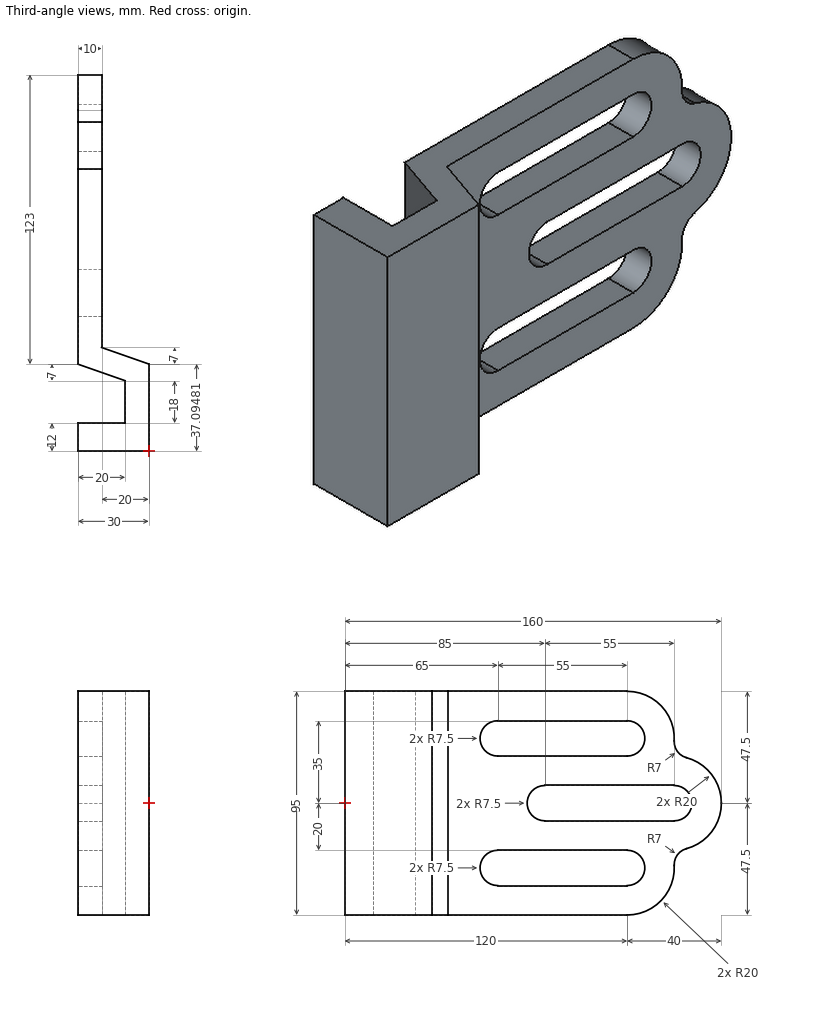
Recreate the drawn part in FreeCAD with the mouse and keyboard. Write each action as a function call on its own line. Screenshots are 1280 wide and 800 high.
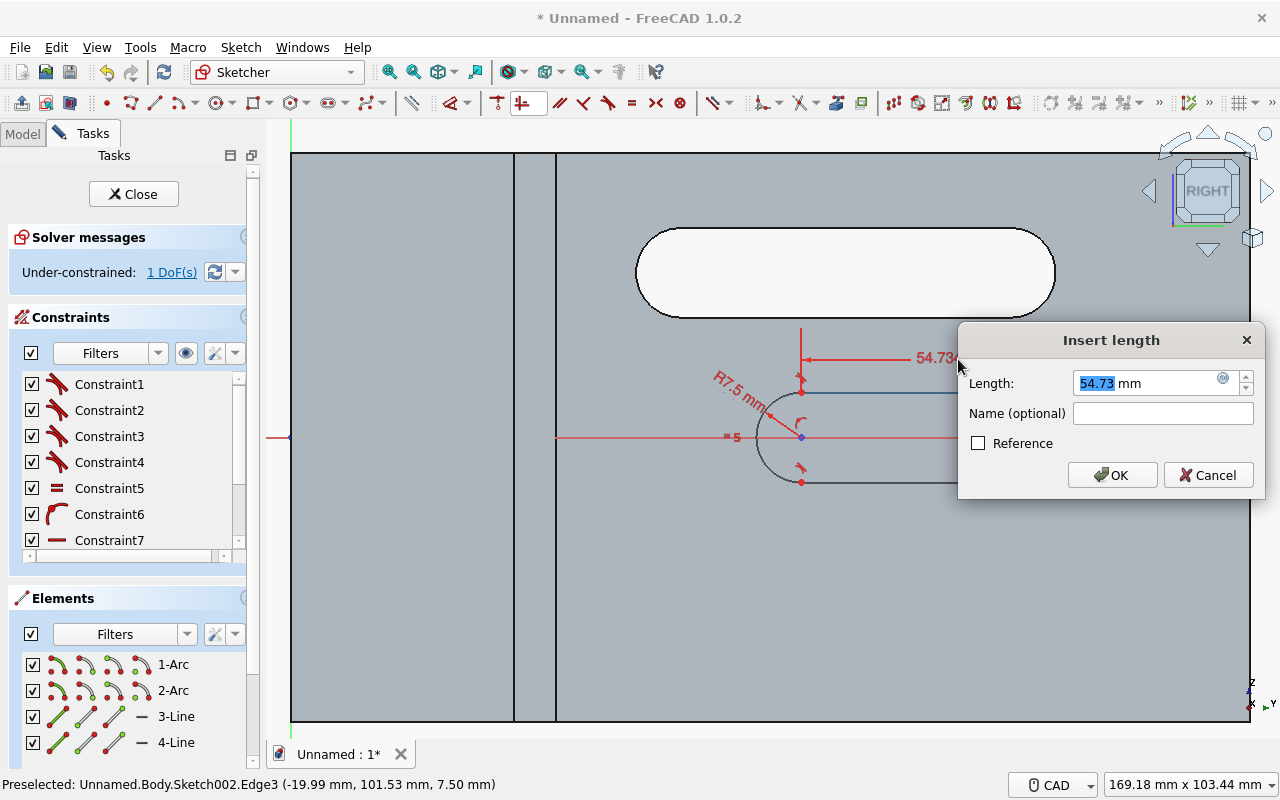
text(55)
key(Return)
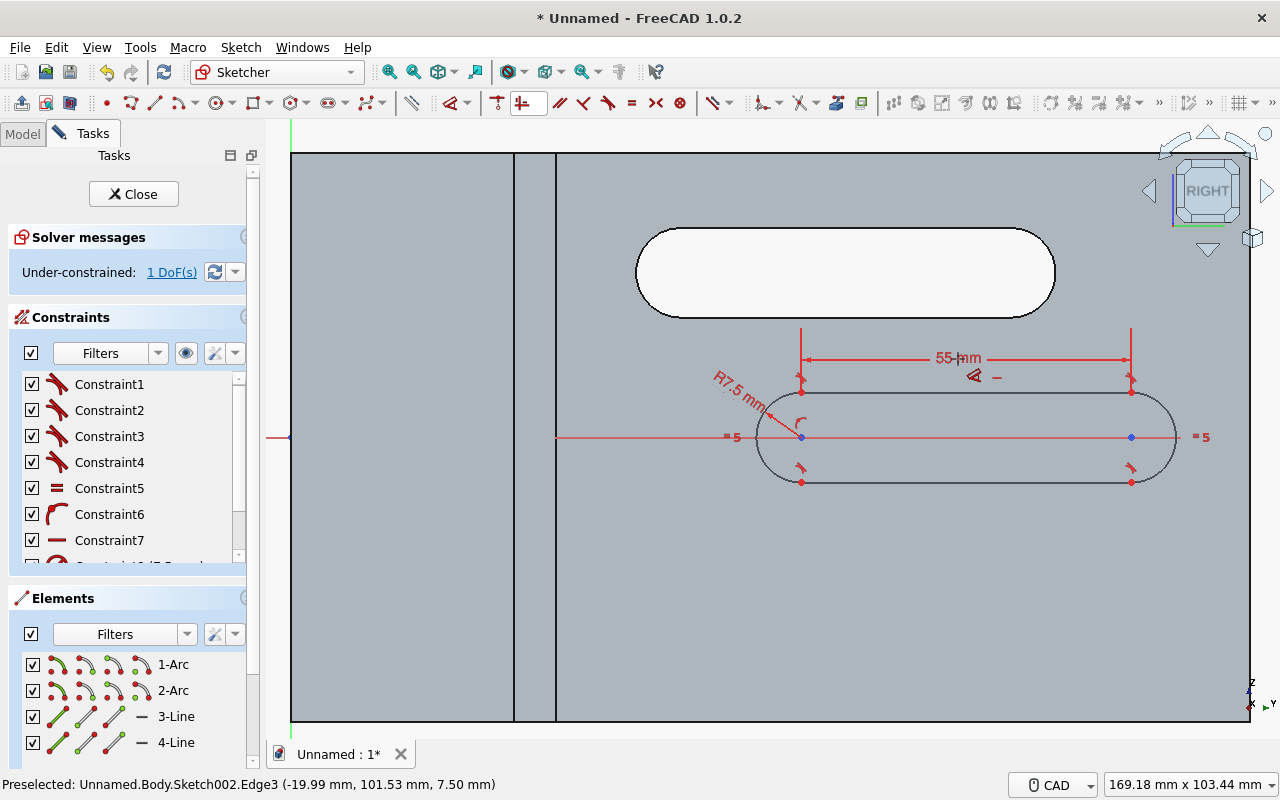
click(801, 393)
click(548, 359)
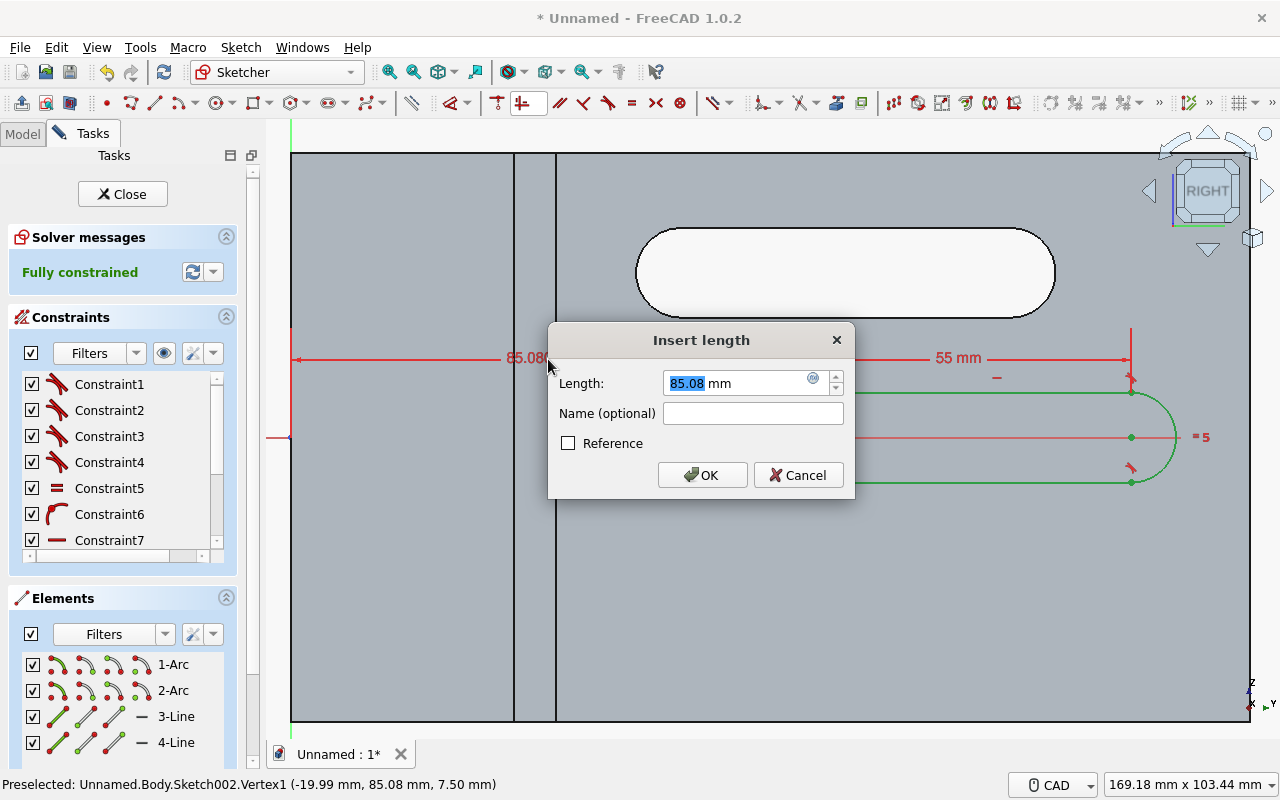
text(85)
key(Return)
key(Escape)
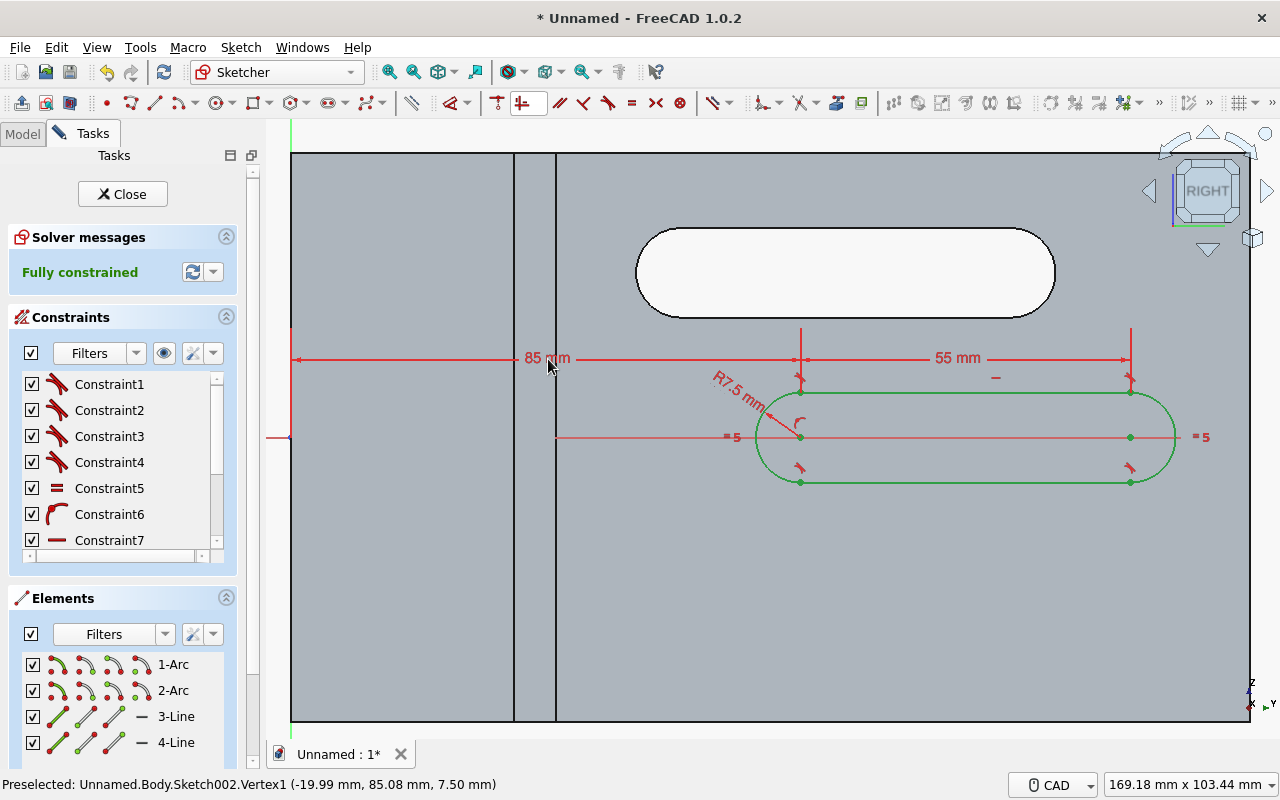
click(123, 194)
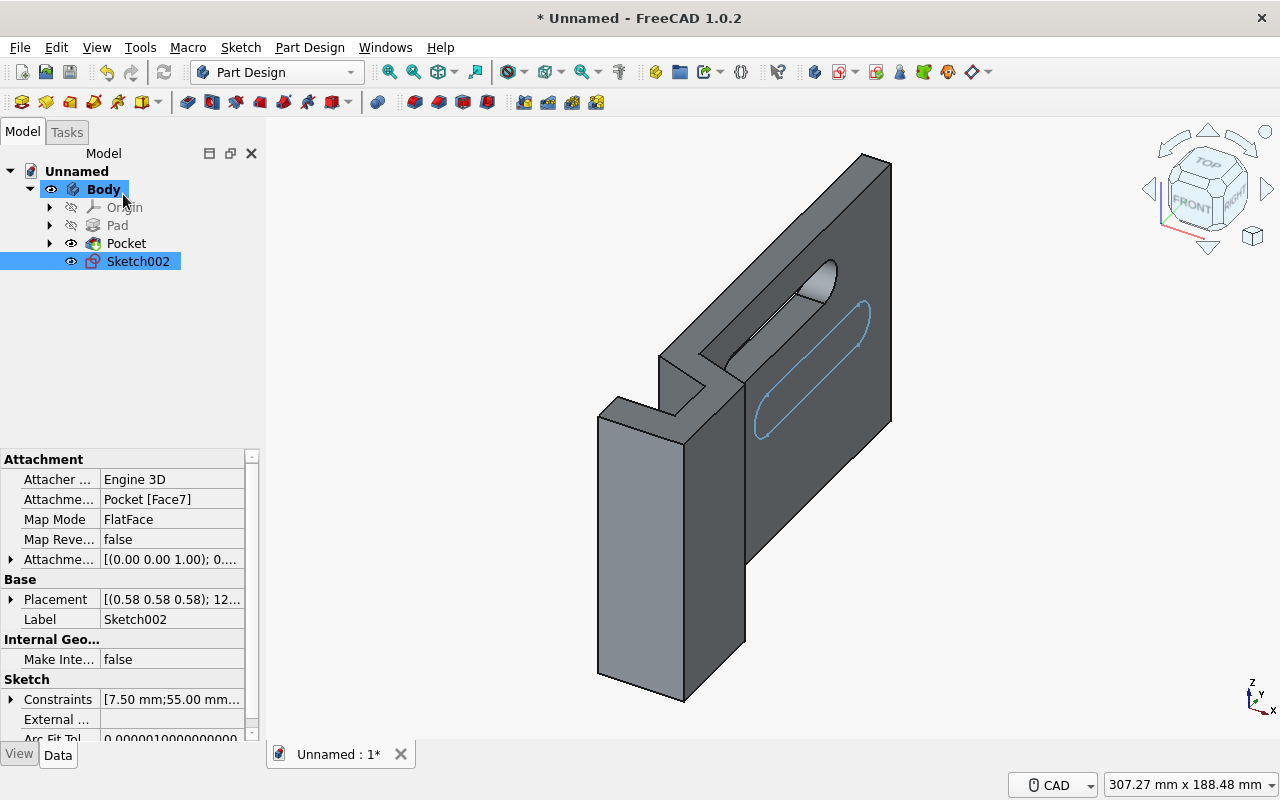
click(188, 102)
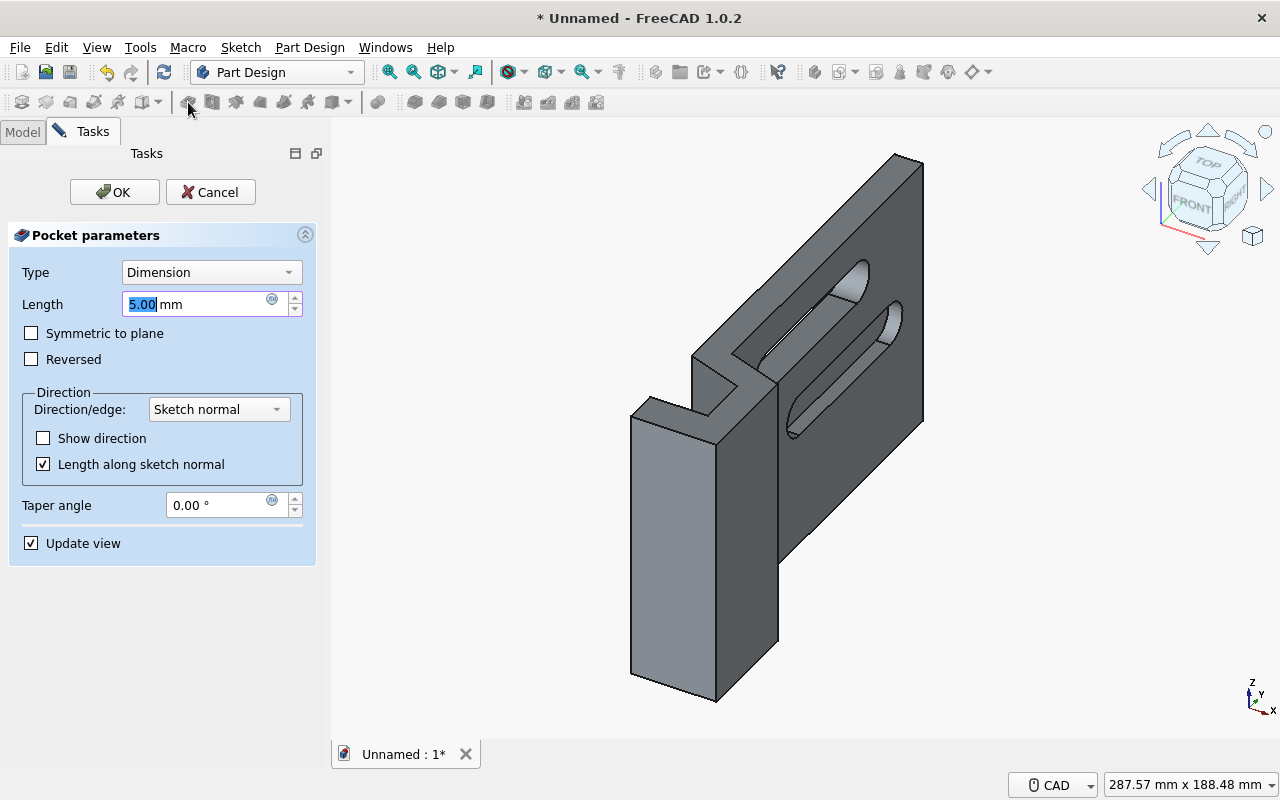
click(212, 272)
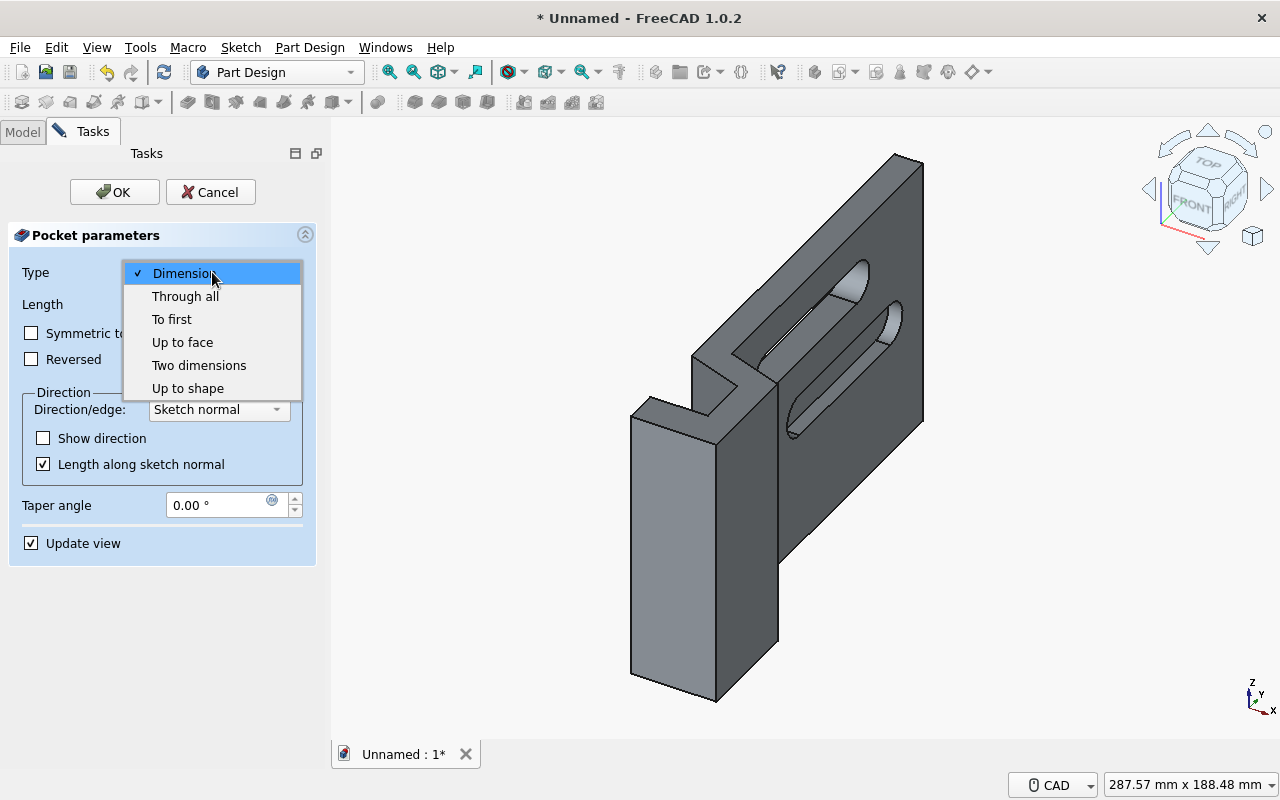
click(212, 320)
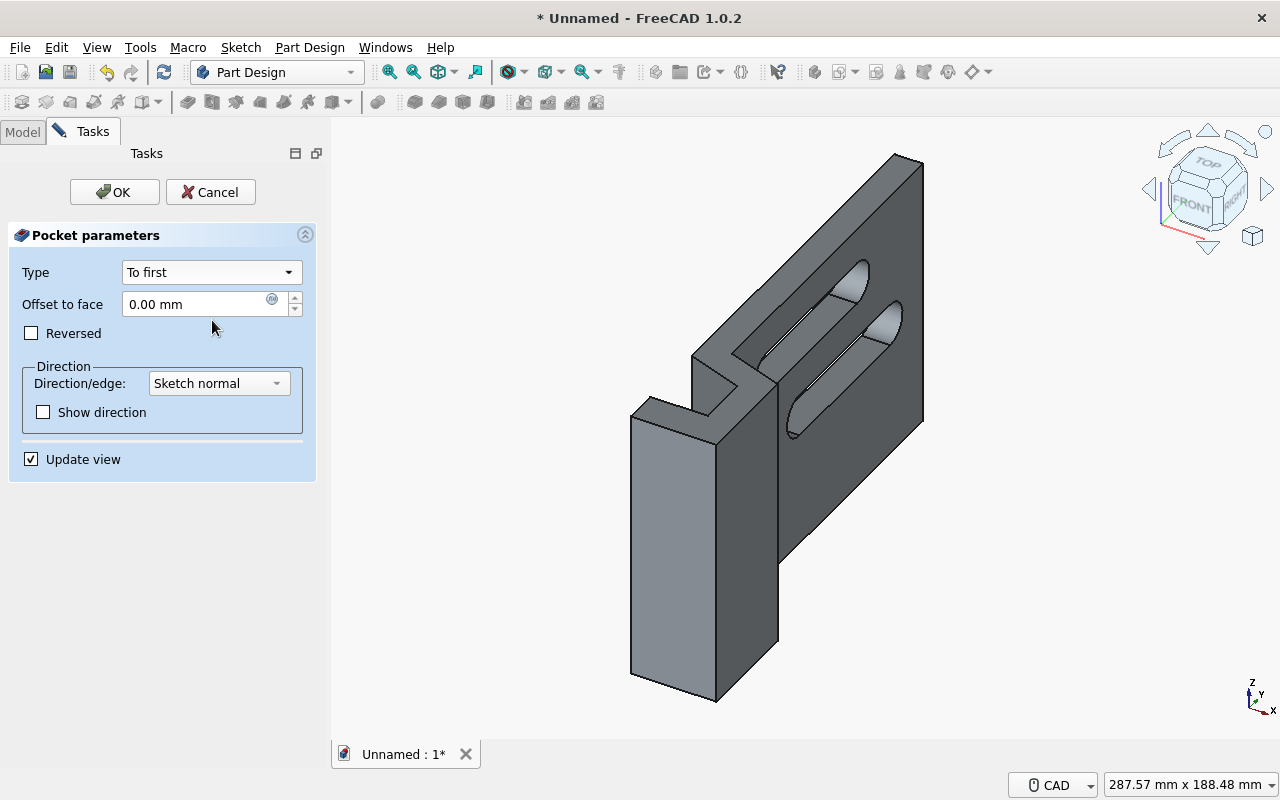
click(115, 192)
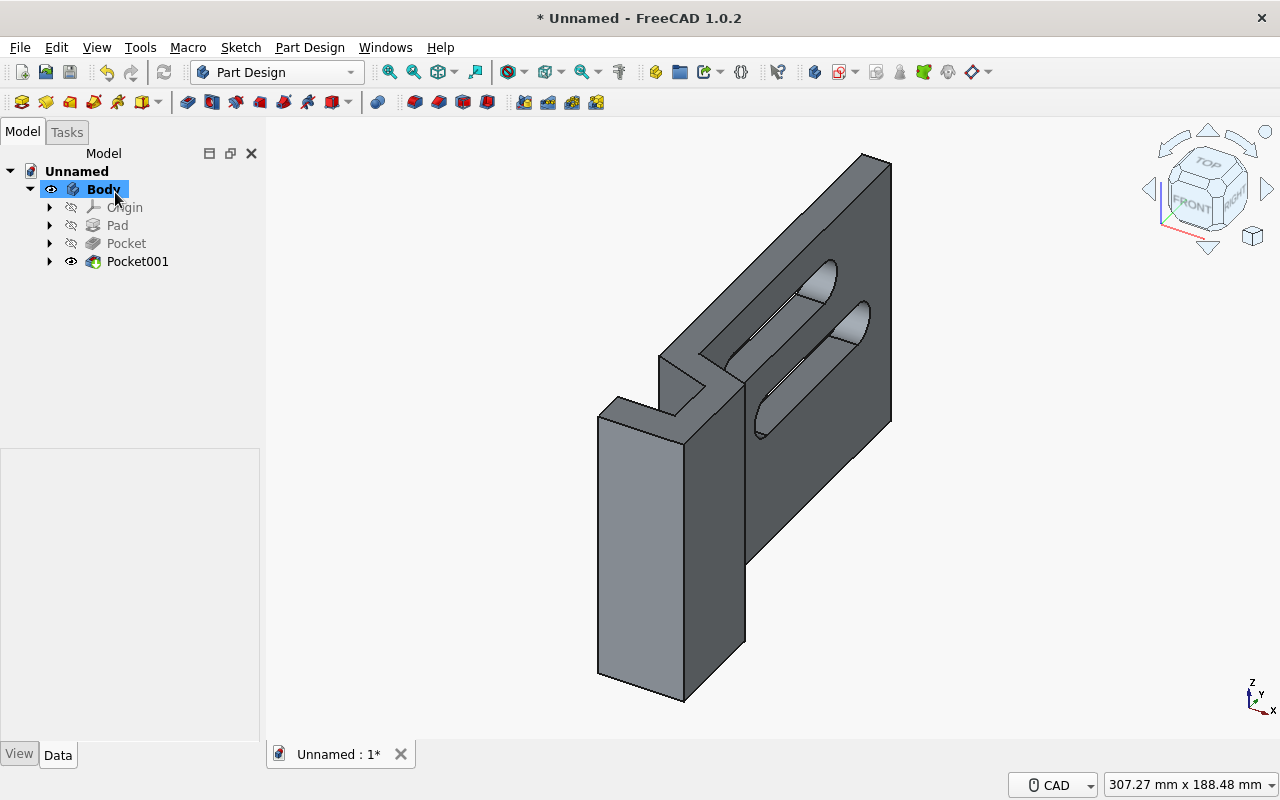
click(850, 405)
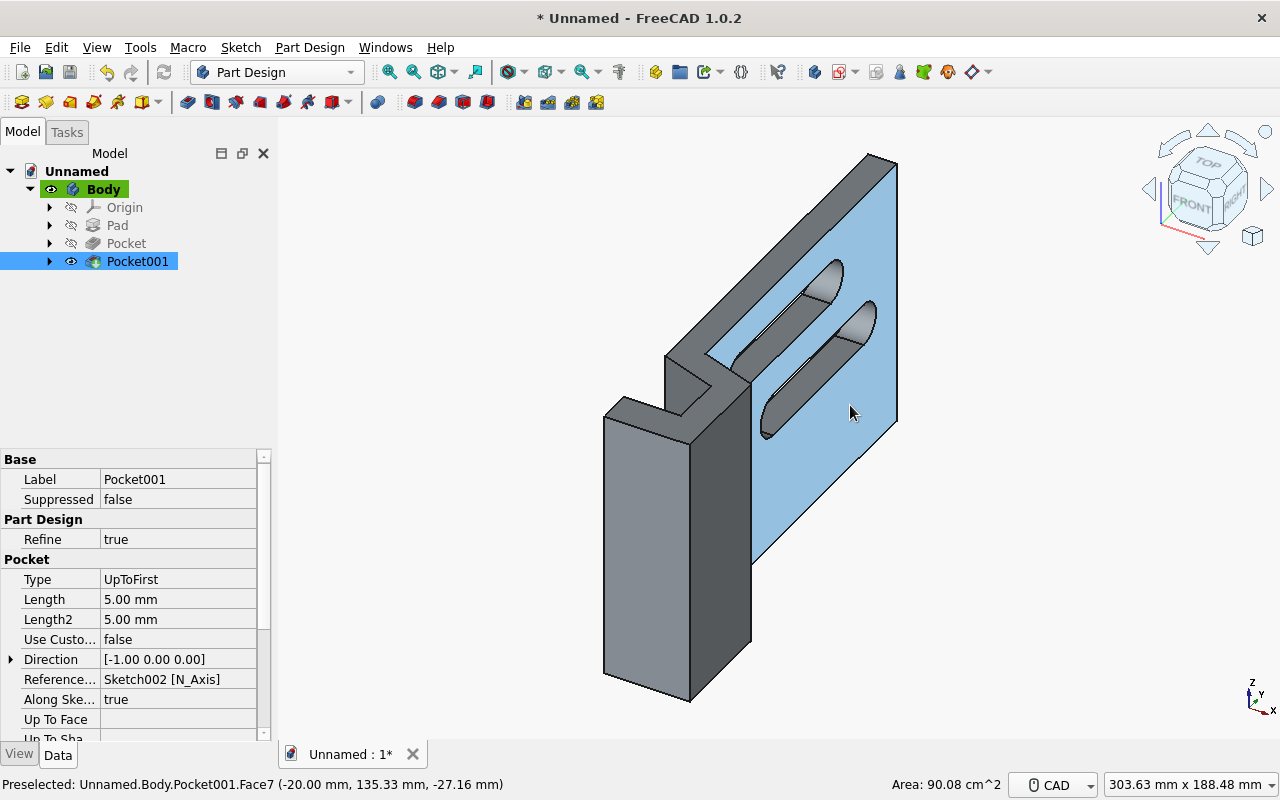
click(840, 72)